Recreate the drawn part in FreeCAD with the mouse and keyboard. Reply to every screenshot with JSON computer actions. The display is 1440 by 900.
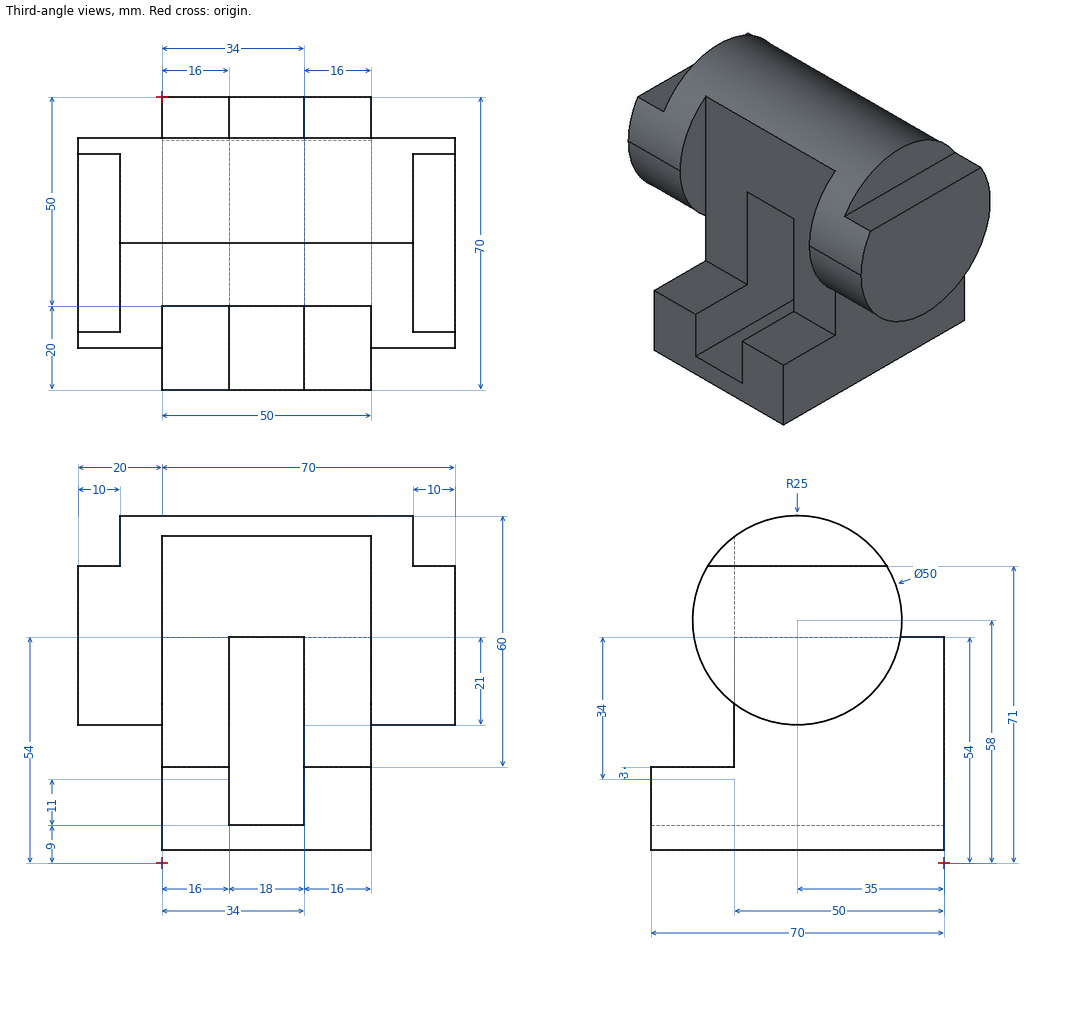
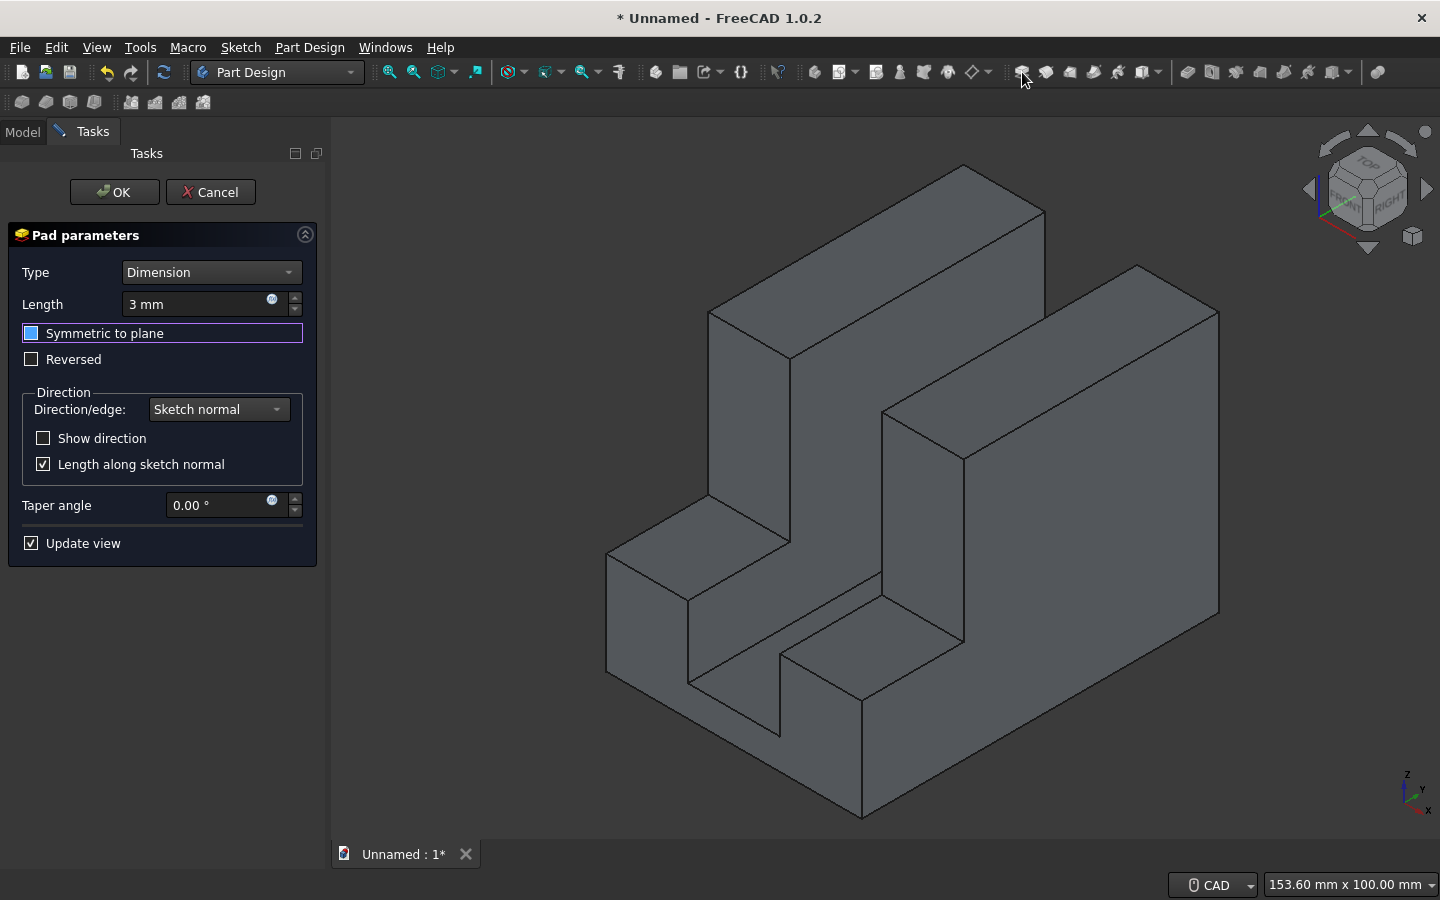
{"action": "left_click", "coordinate": [115, 192]}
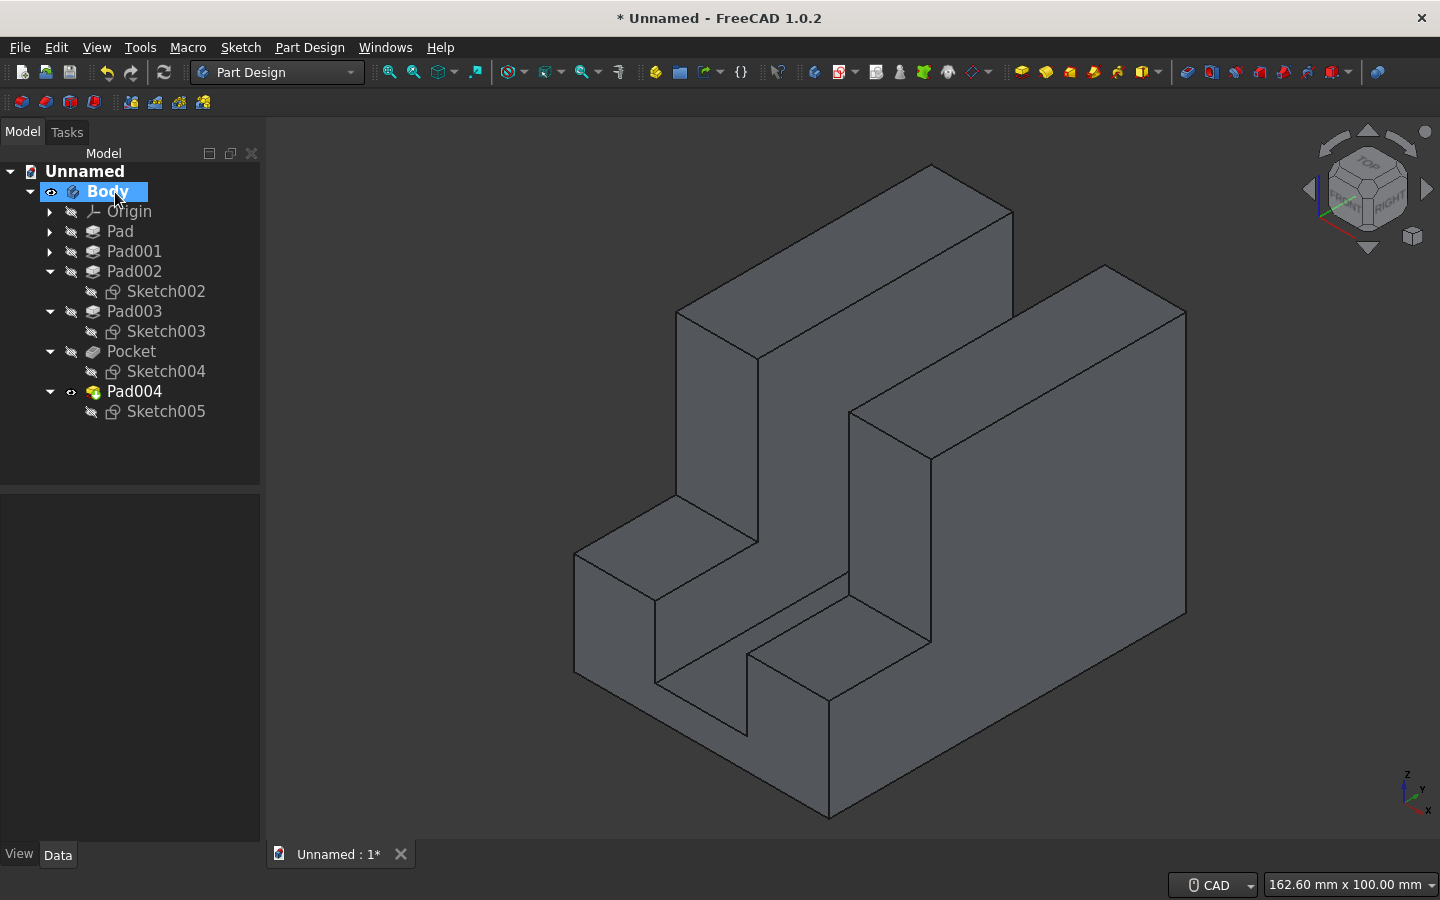
{"action": "key", "text": "6"}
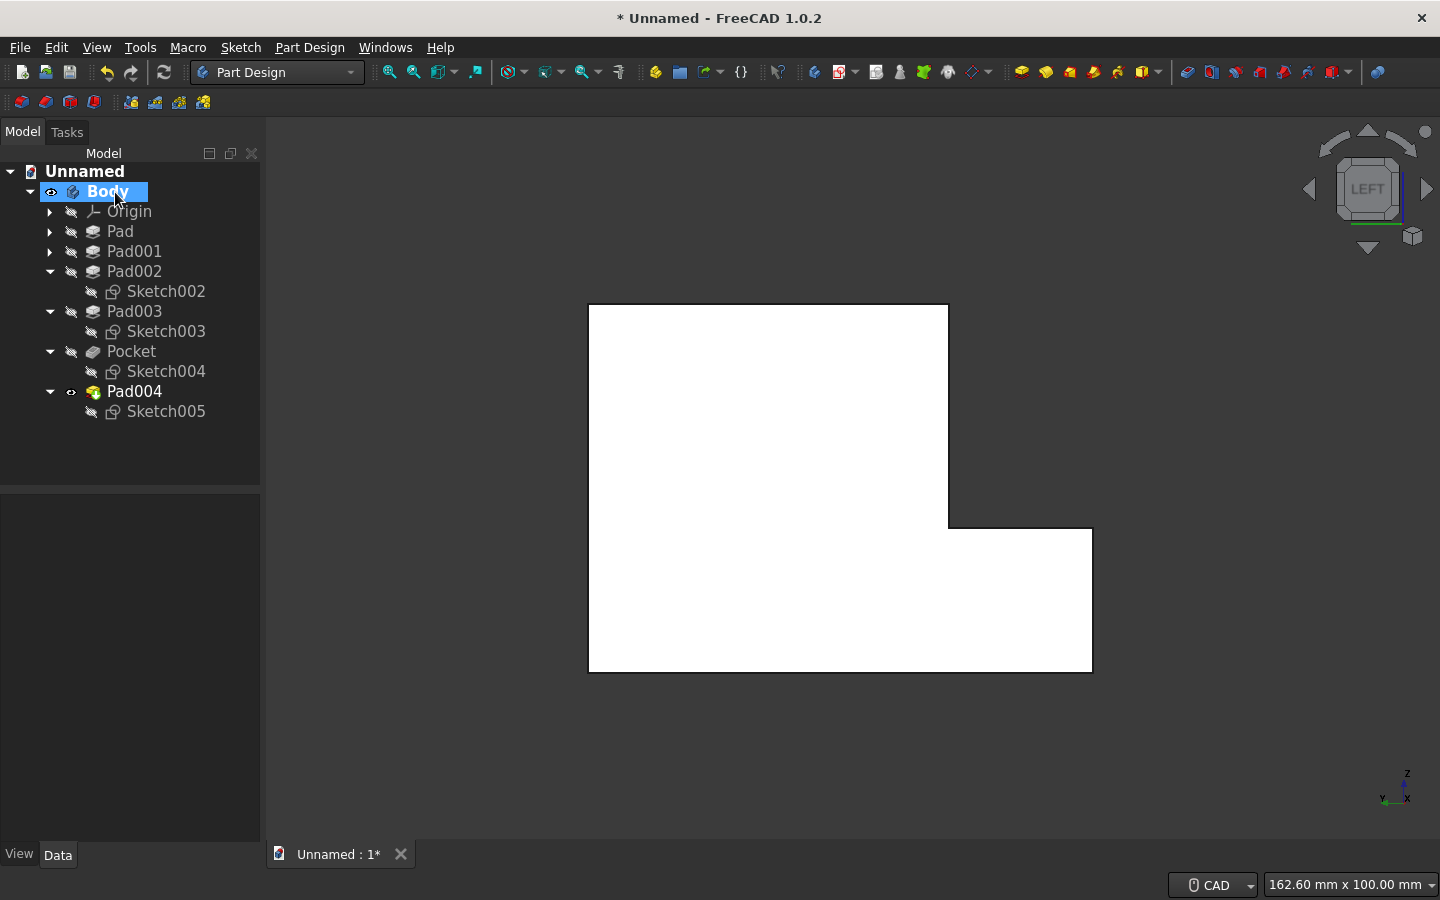
{"action": "left_click", "coordinate": [768, 488]}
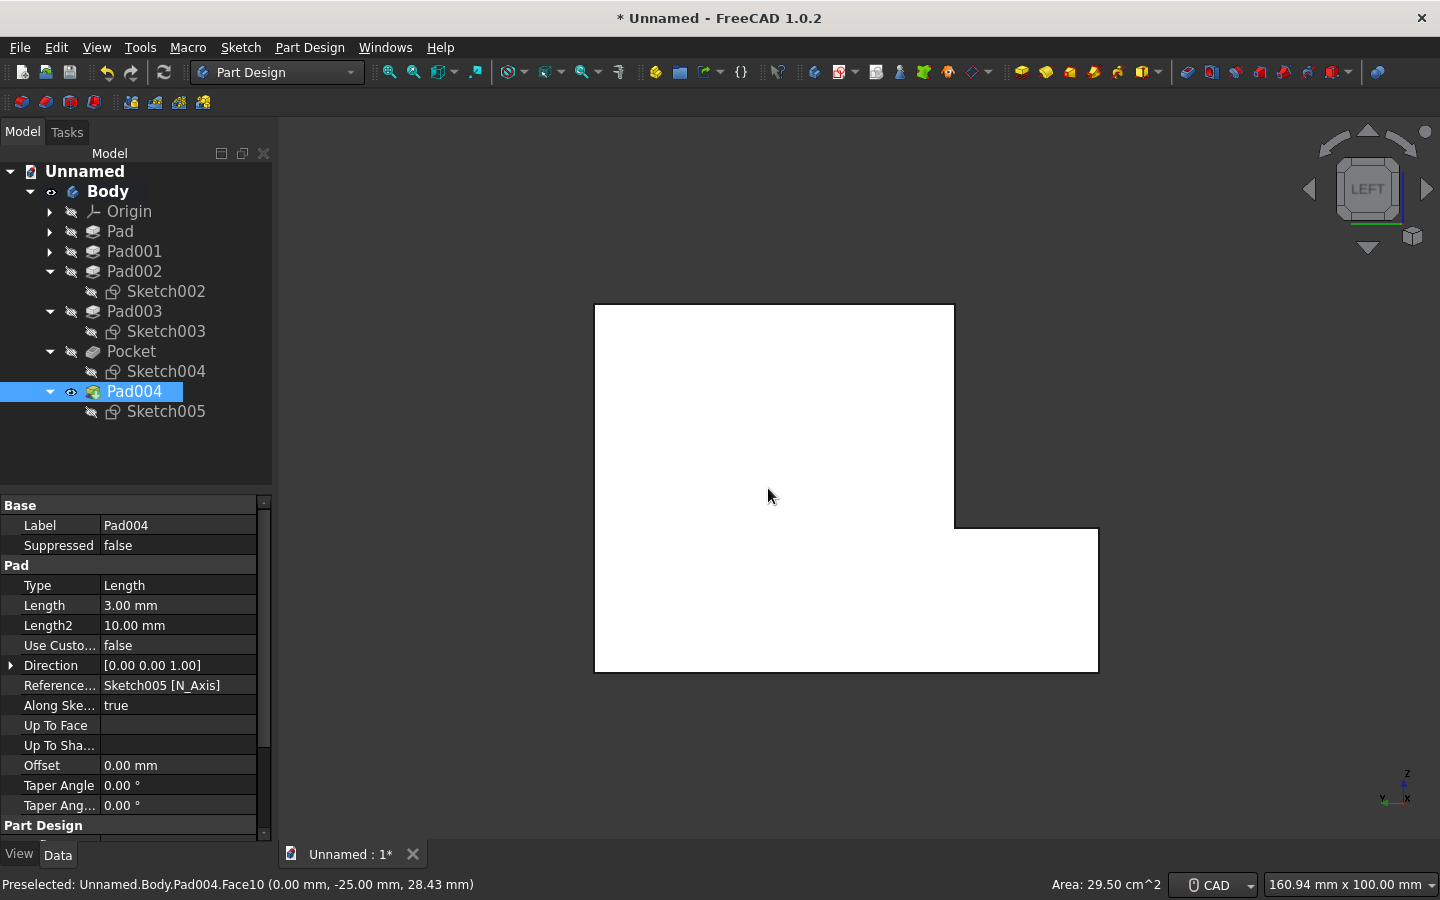
{"action": "left_click", "coordinate": [840, 72]}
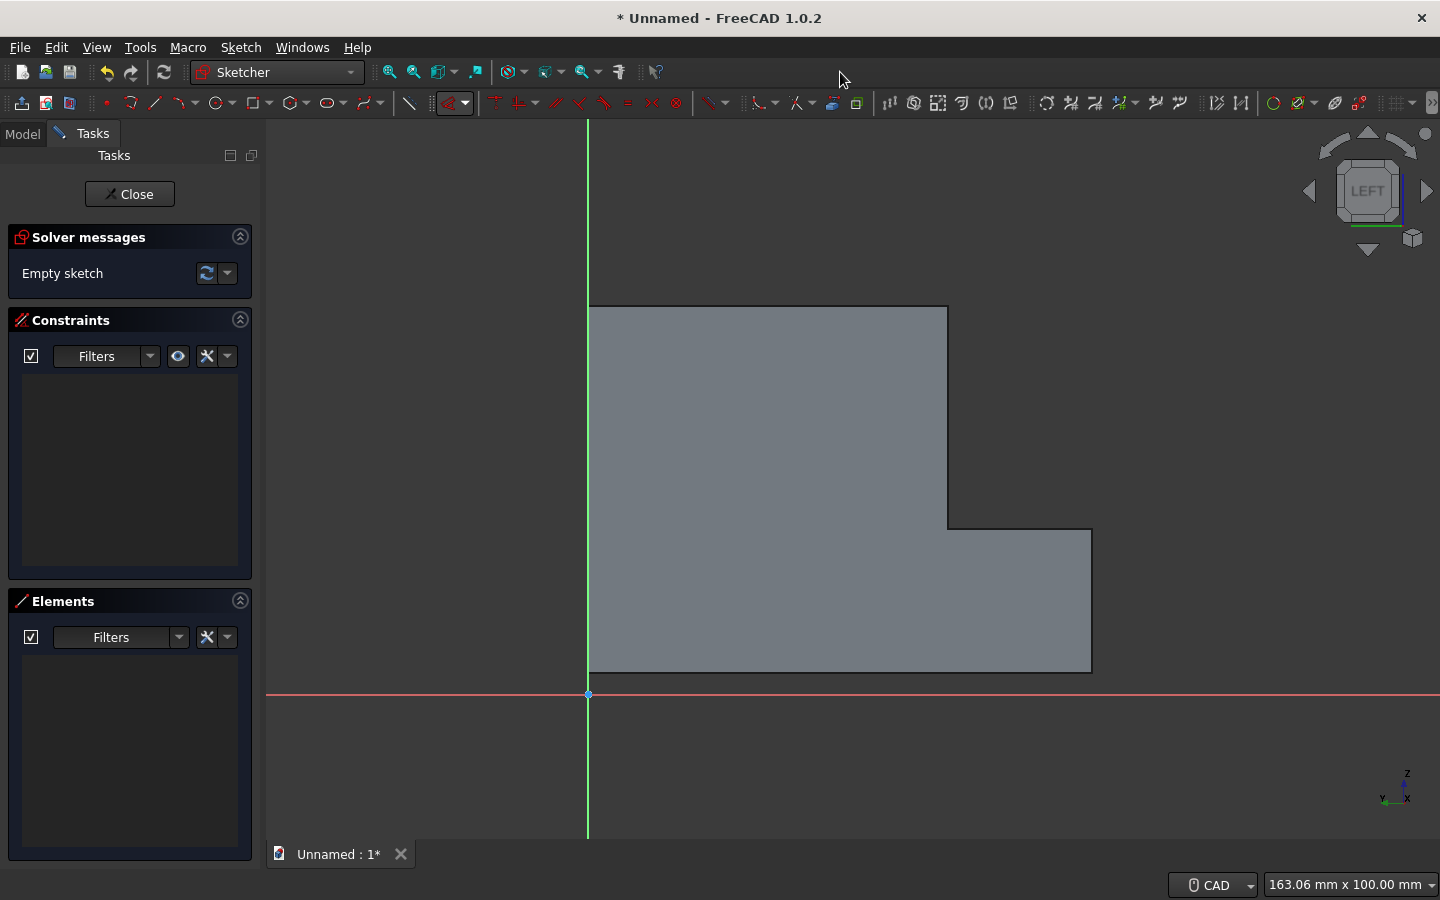
{"action": "scroll", "coordinate": [695, 811], "scroll_direction": "down", "scroll_amount": 1}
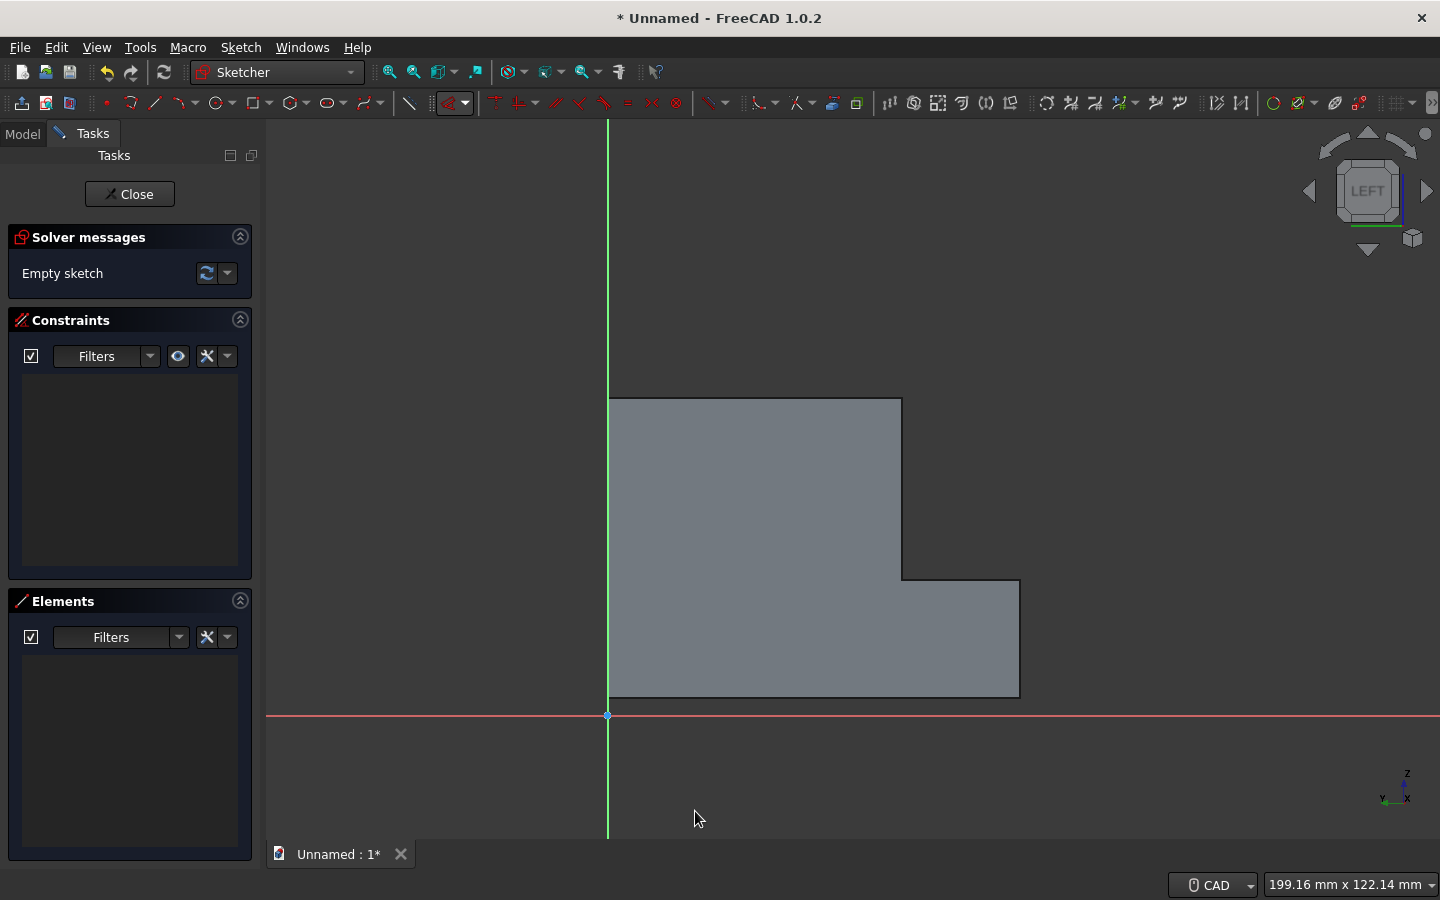
{"action": "key", "text": "g c"}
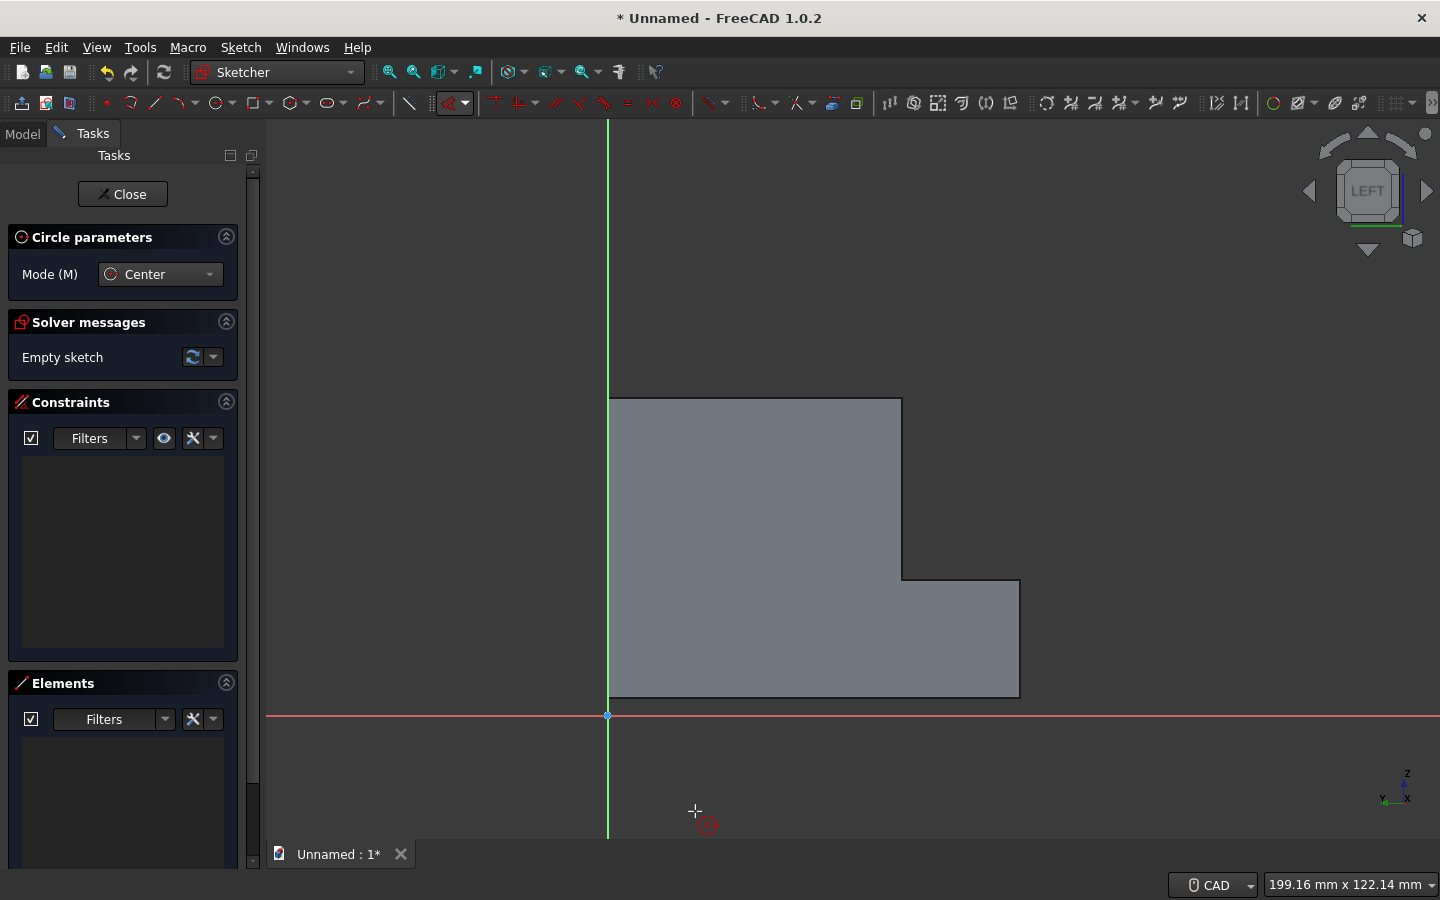
{"action": "left_click", "coordinate": [814, 374]}
{"action": "mouse_move", "coordinate": [918, 270]}